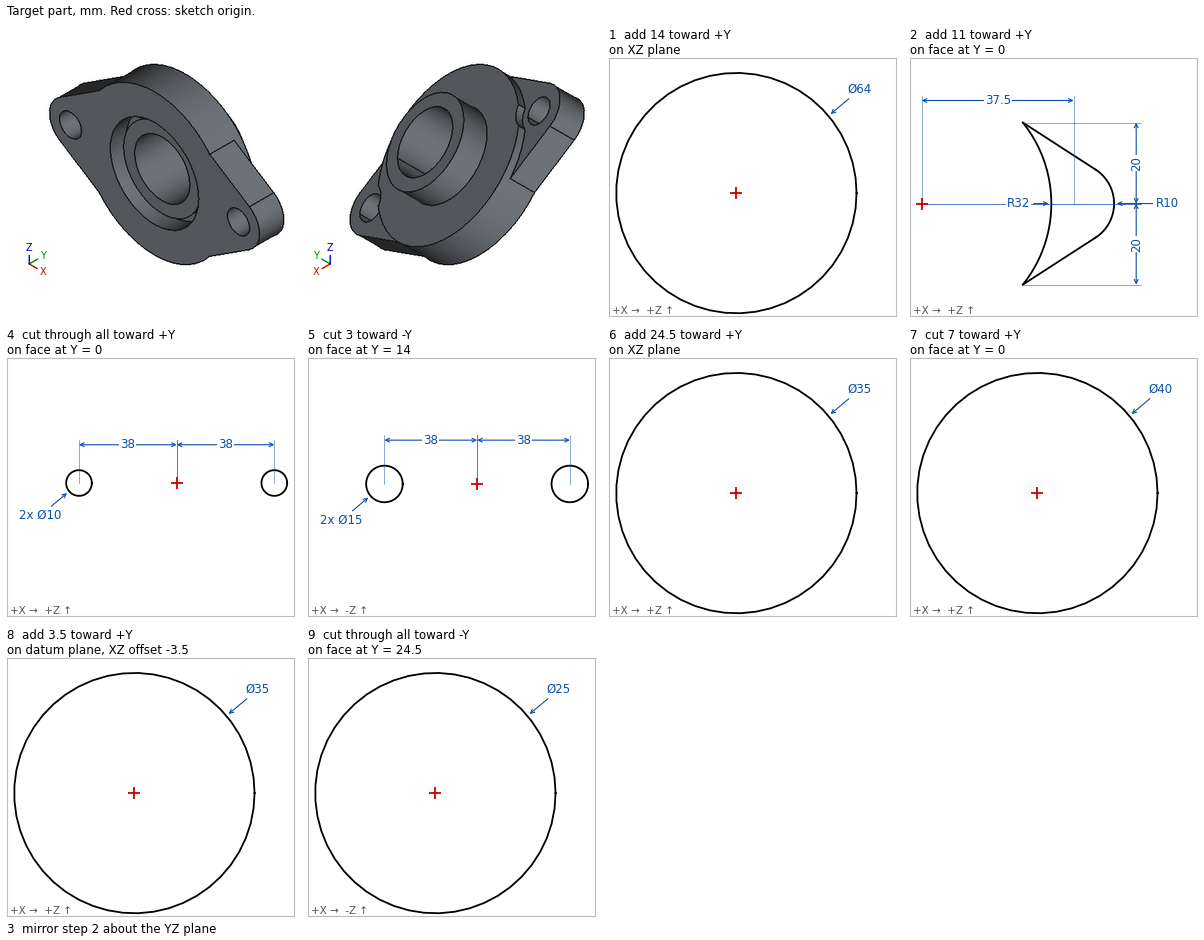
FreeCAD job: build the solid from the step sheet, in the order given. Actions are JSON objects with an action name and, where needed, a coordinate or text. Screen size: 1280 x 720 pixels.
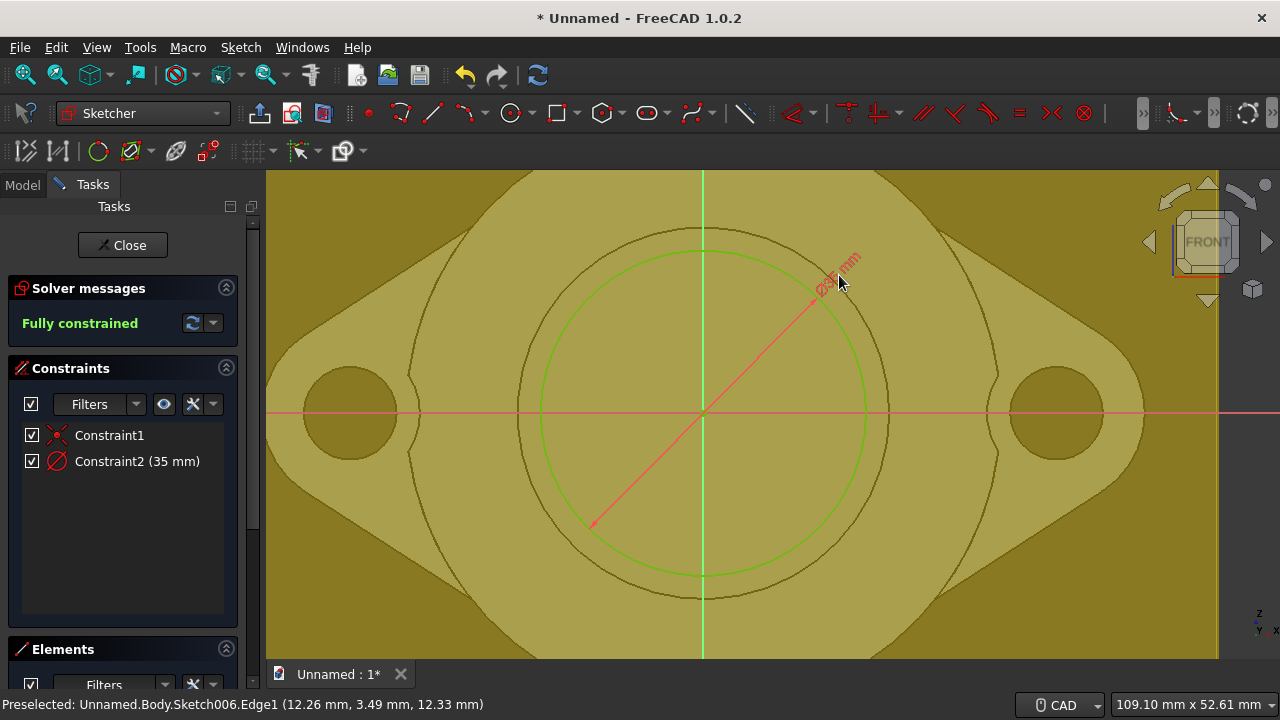
{"action": "left_click", "coordinate": [123, 245]}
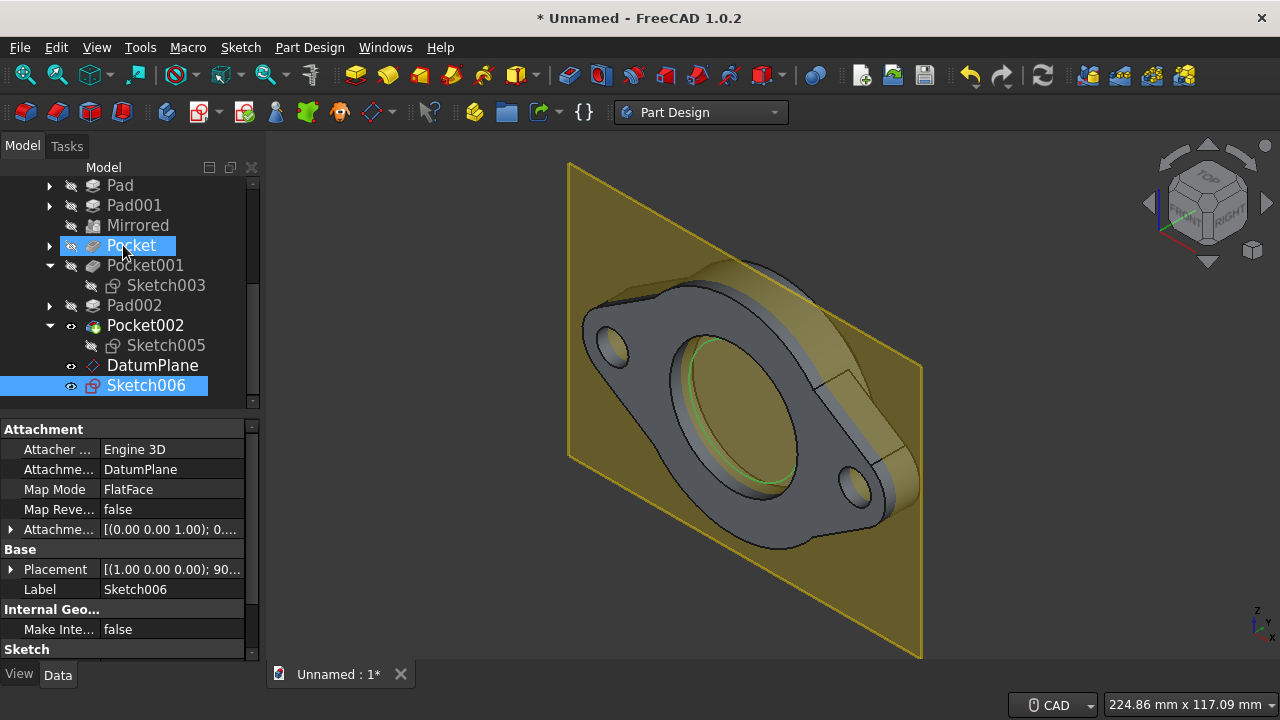
{"action": "left_click", "coordinate": [356, 76]}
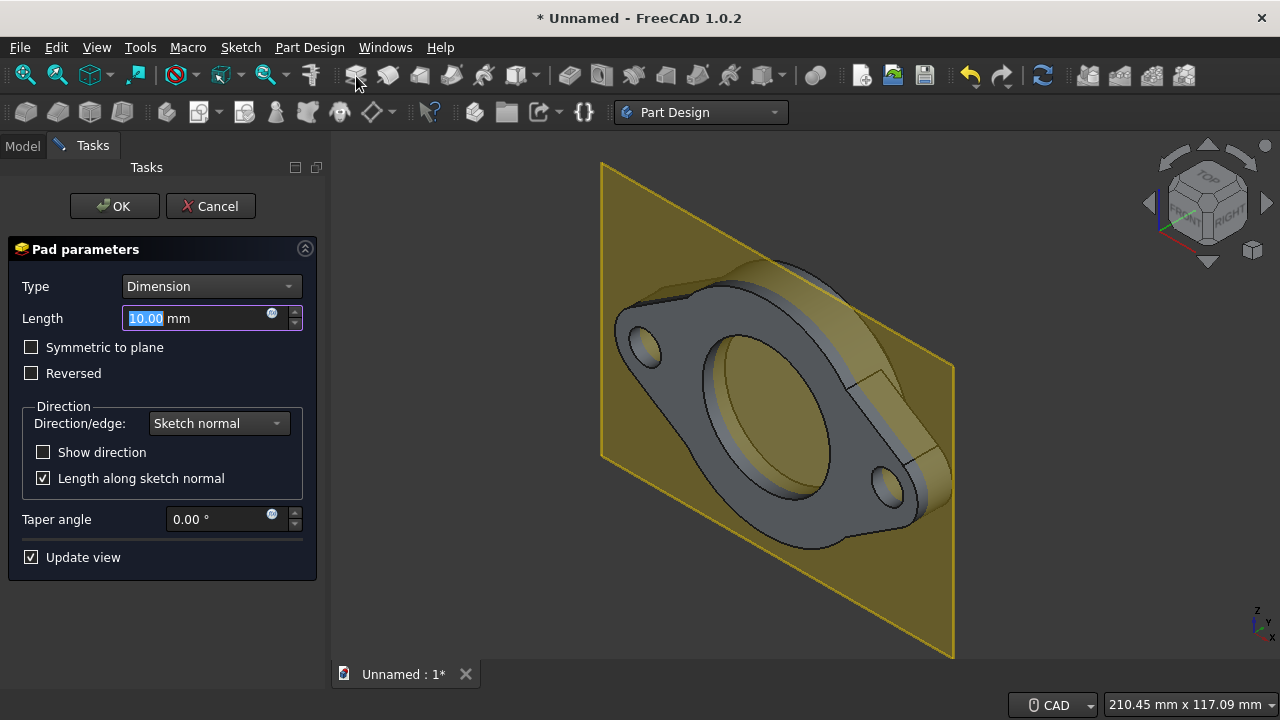
{"action": "type", "text": "3.5"}
{"action": "key", "text": "Tab"}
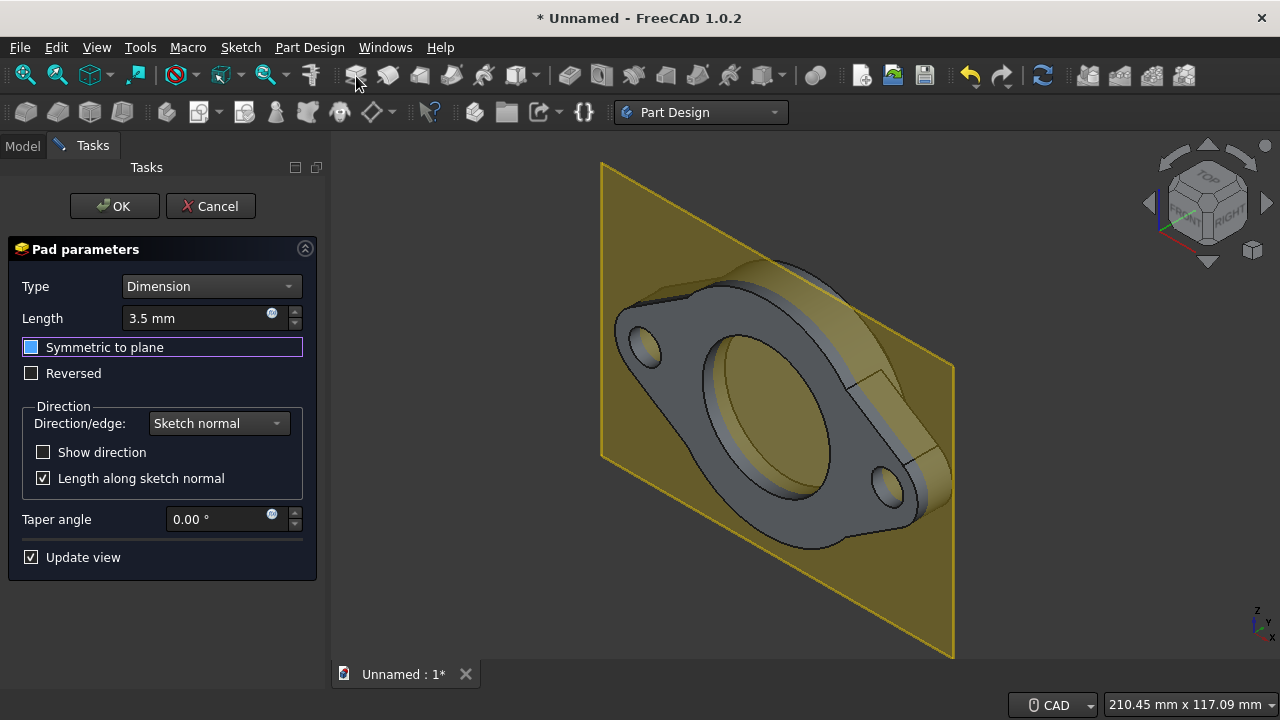
{"action": "left_click", "coordinate": [30, 373]}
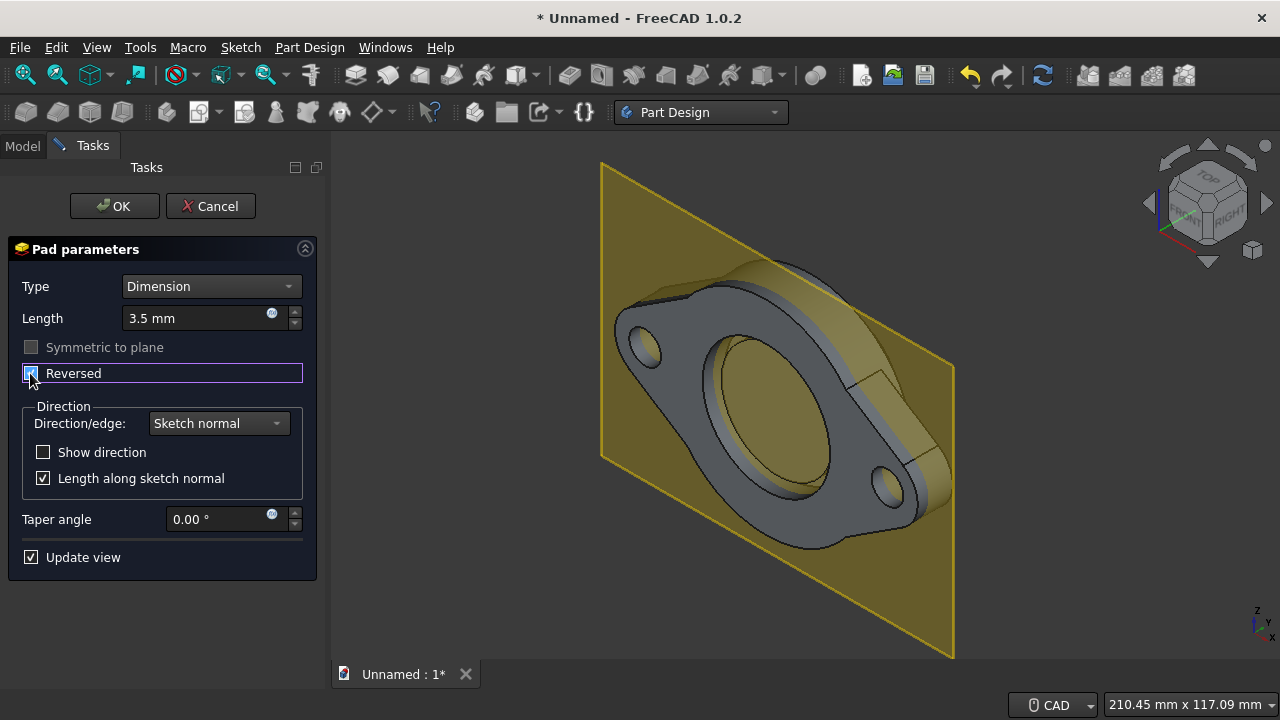
{"action": "left_click", "coordinate": [115, 206]}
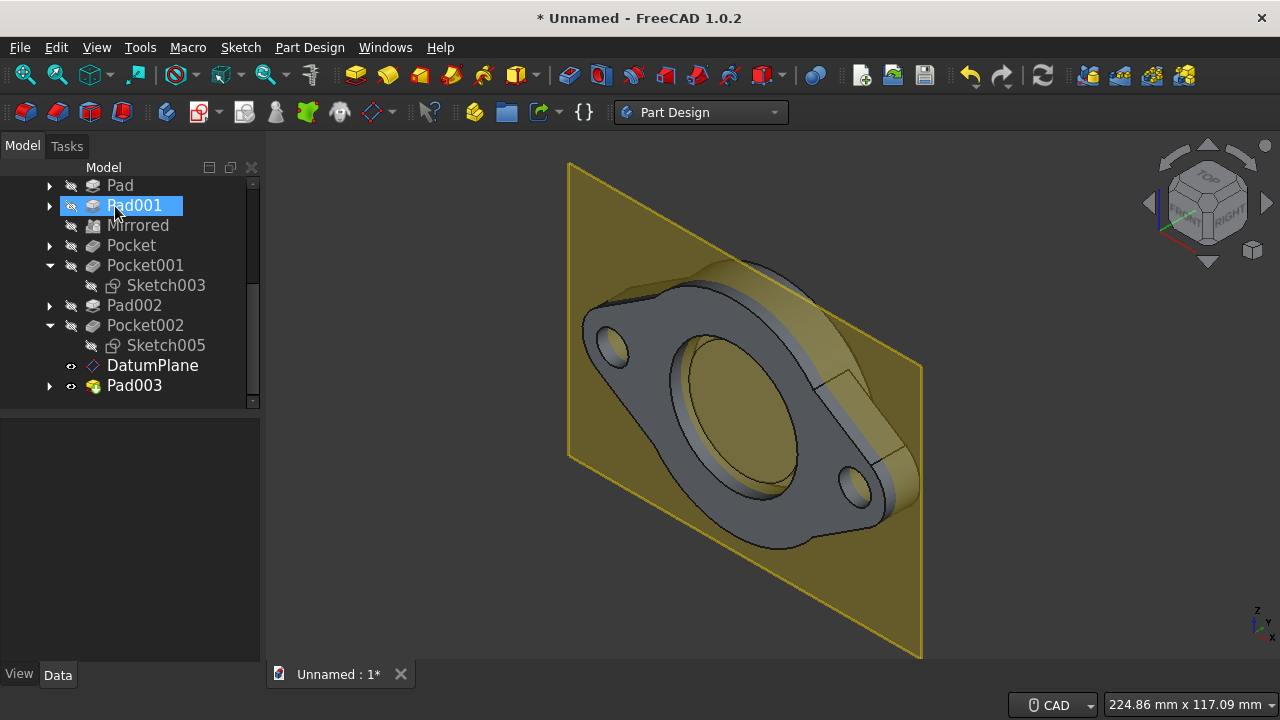
{"action": "left_click", "coordinate": [116, 366]}
{"action": "key", "text": "space"}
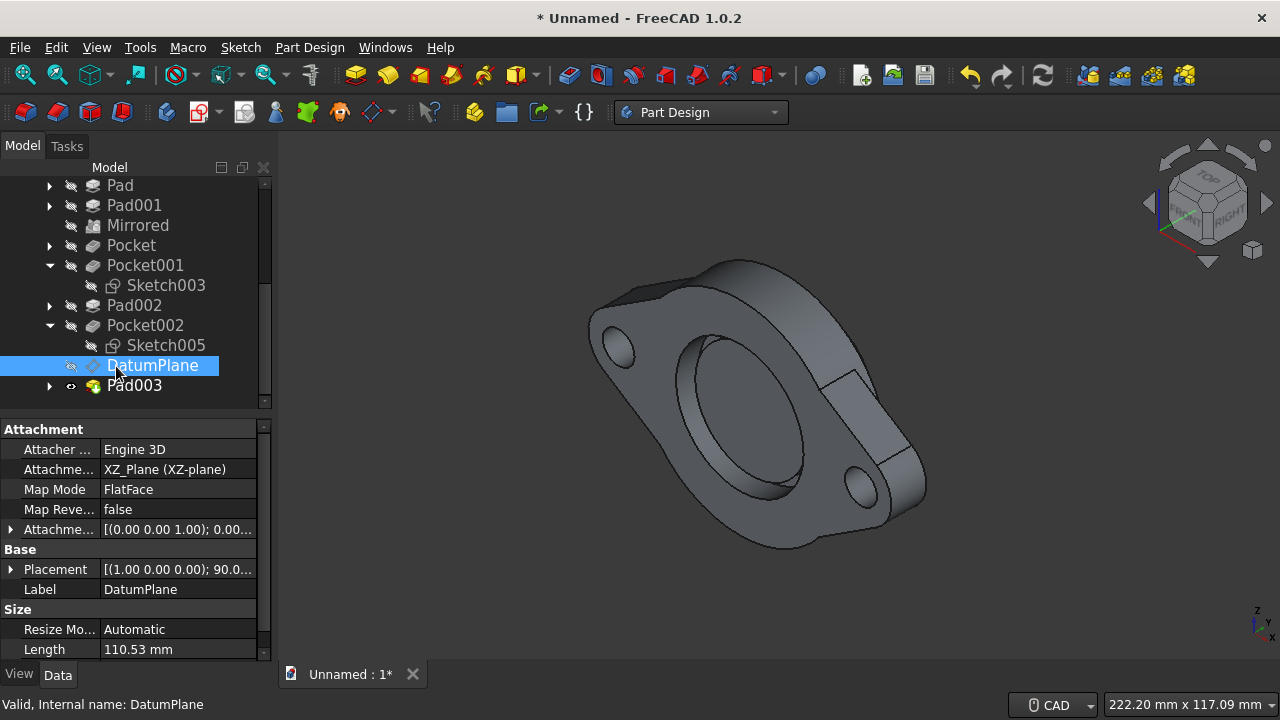
{"action": "key", "text": "4"}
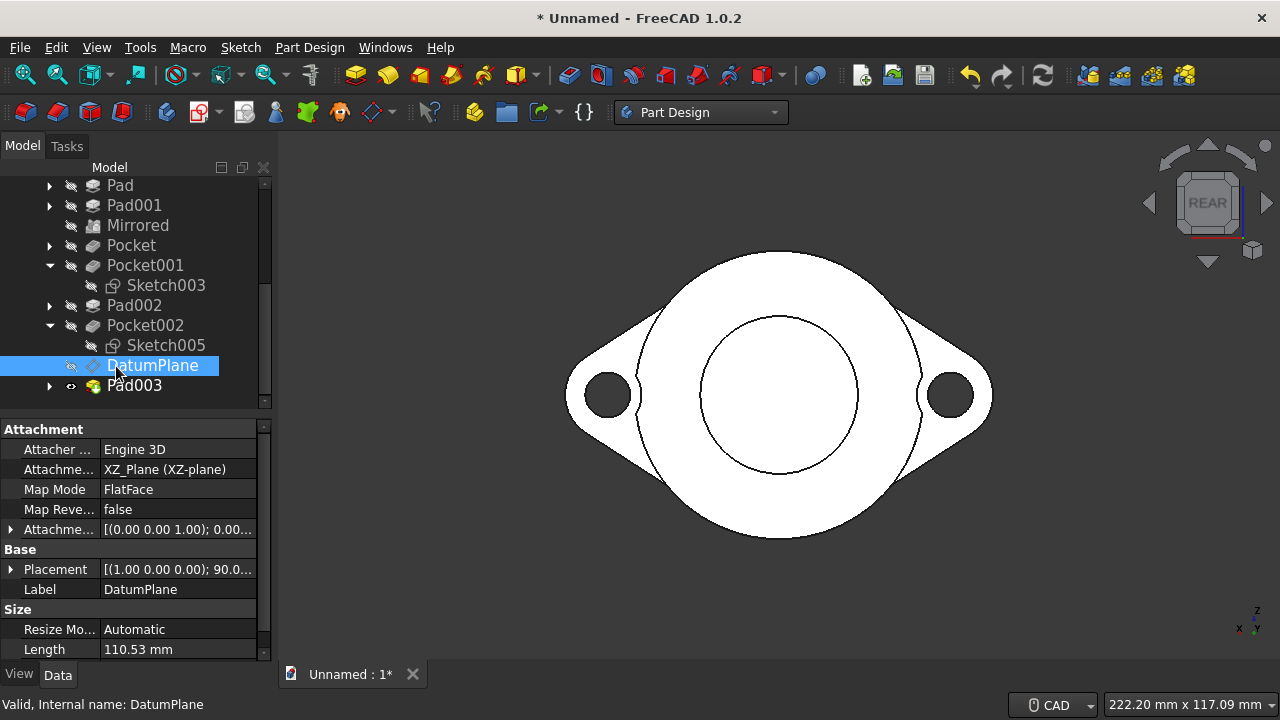
{"action": "left_click", "coordinate": [779, 394]}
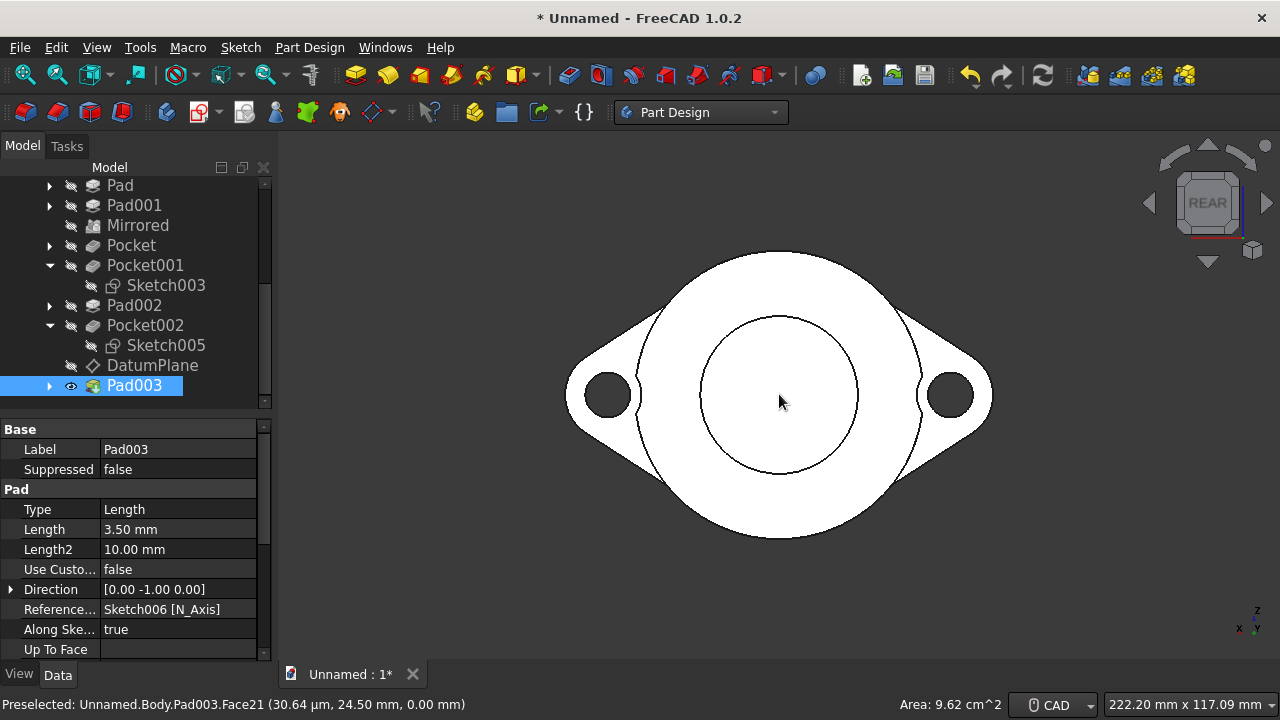
{"action": "left_click", "coordinate": [200, 112]}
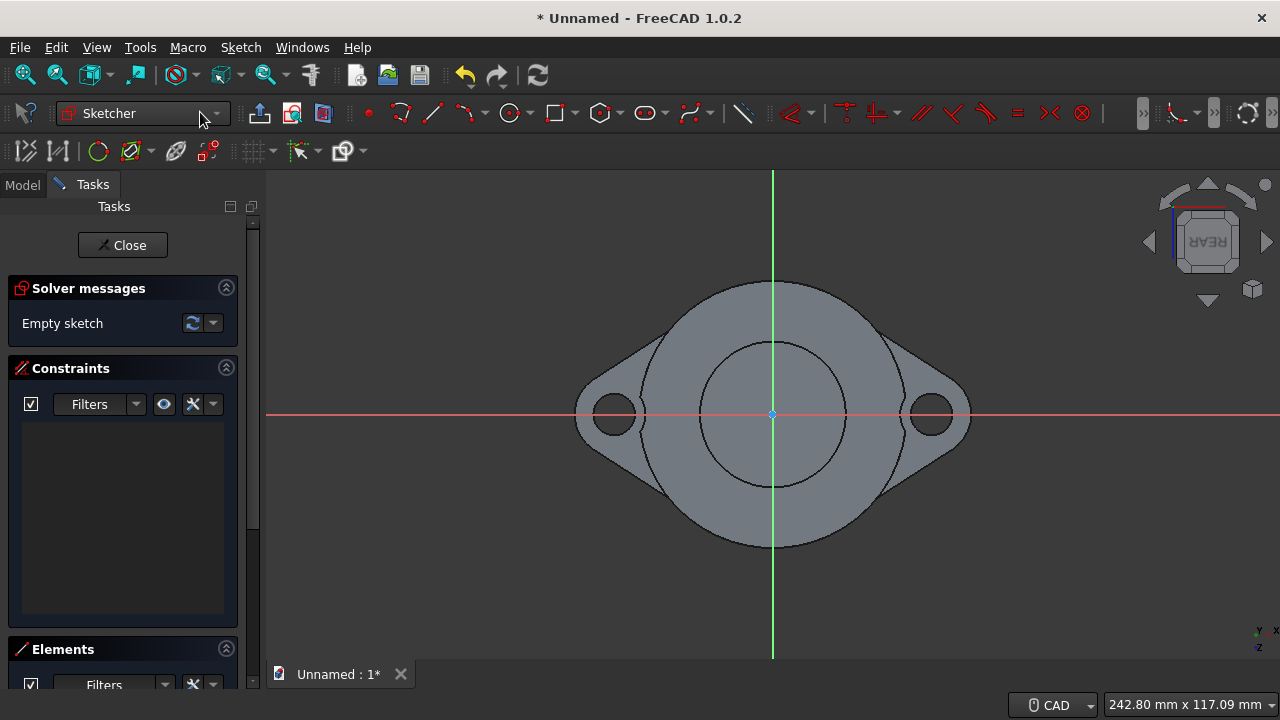
{"action": "scroll", "coordinate": [813, 415], "scroll_direction": "up", "scroll_amount": 5}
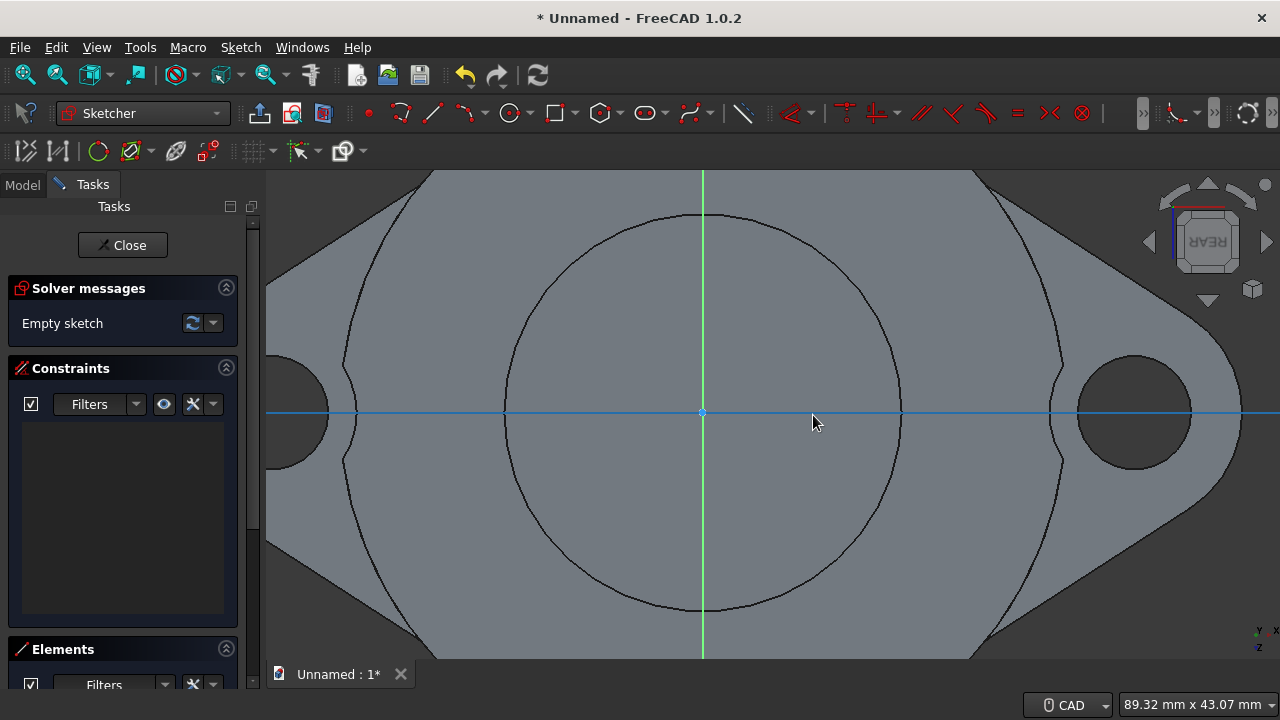
{"action": "left_click", "coordinate": [510, 114]}